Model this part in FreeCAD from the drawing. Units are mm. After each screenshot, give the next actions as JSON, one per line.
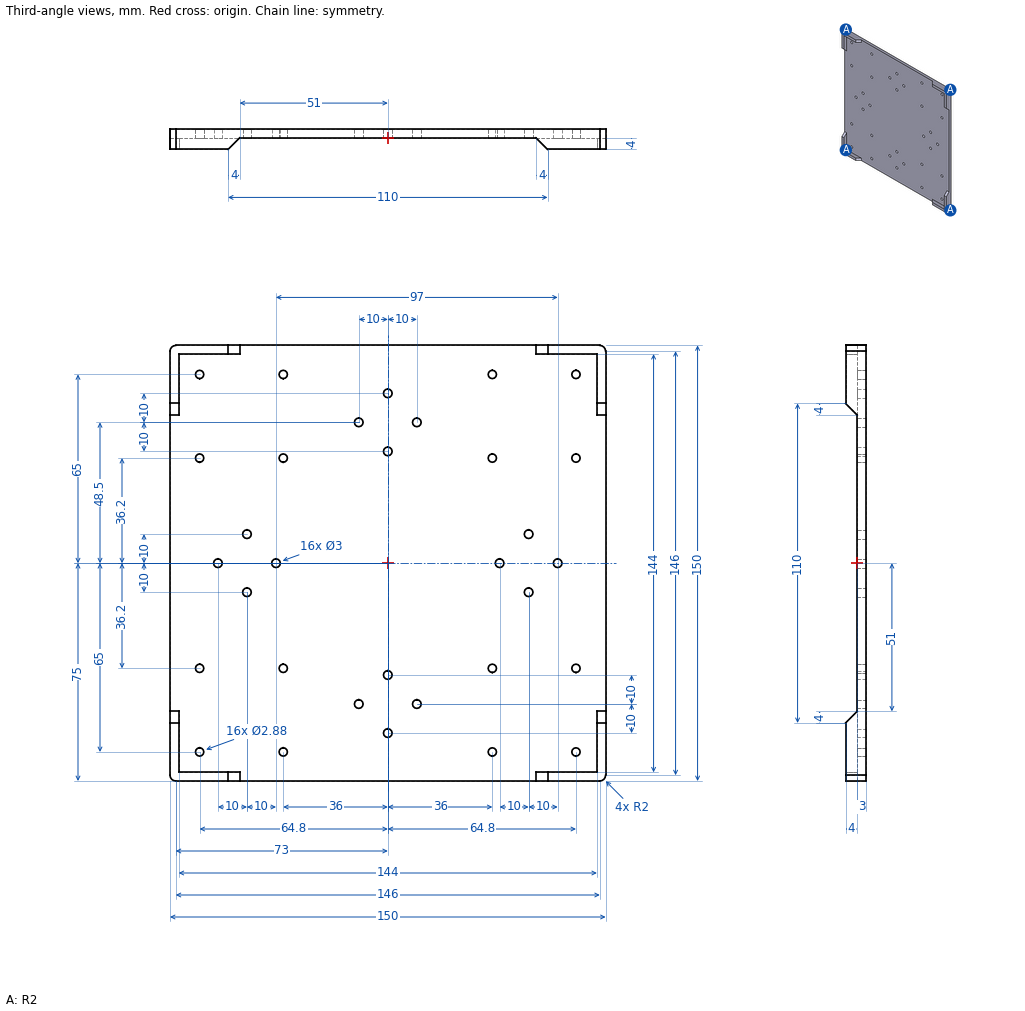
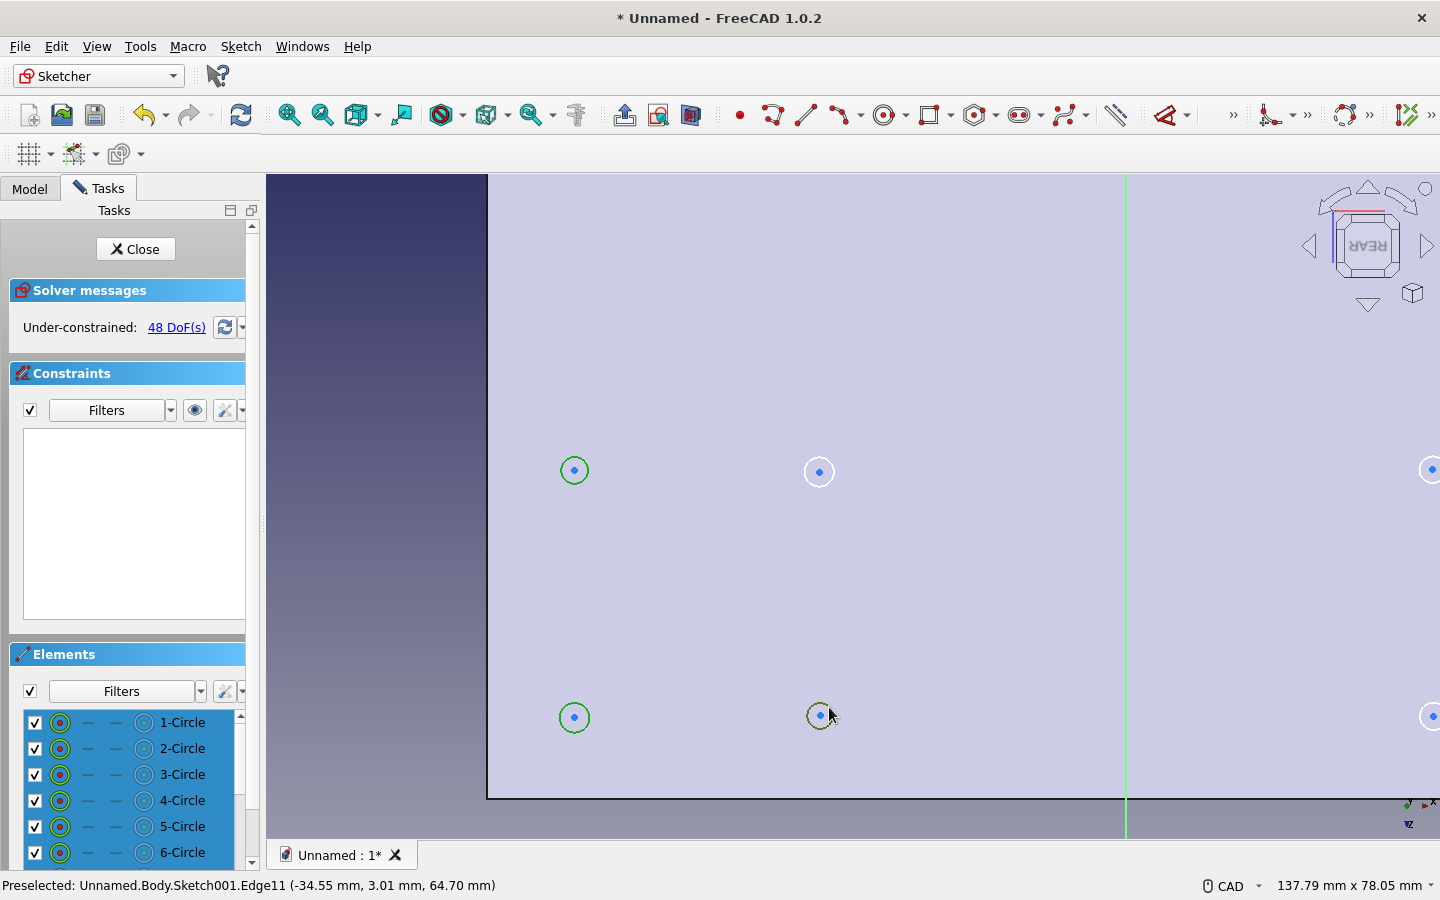
{"action": "left_click", "coordinate": [830, 462]}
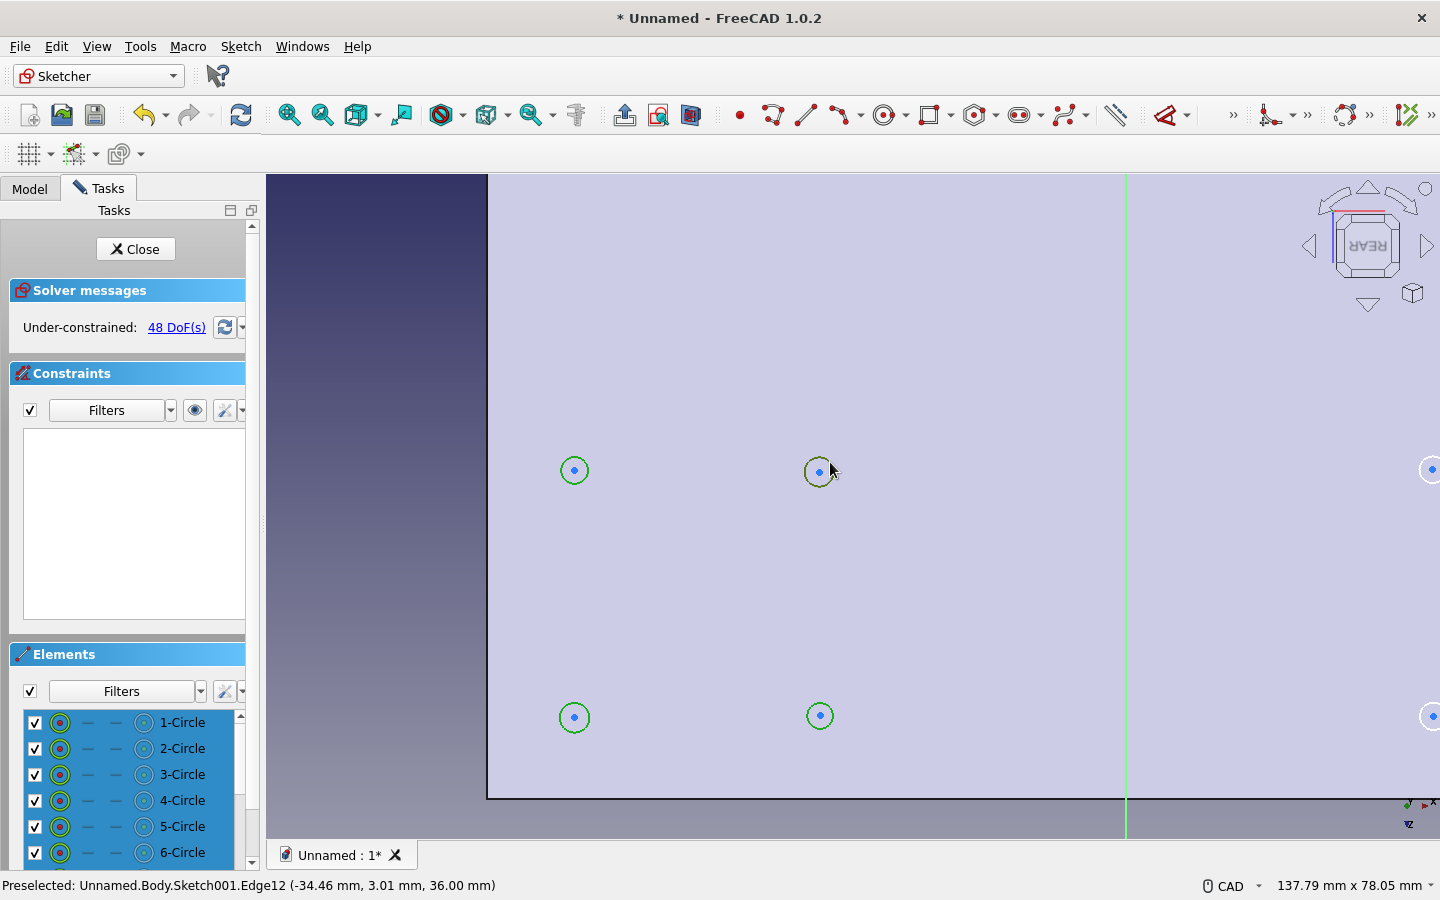
{"action": "scroll", "coordinate": [585, 708], "scroll_direction": "down", "scroll_amount": 5}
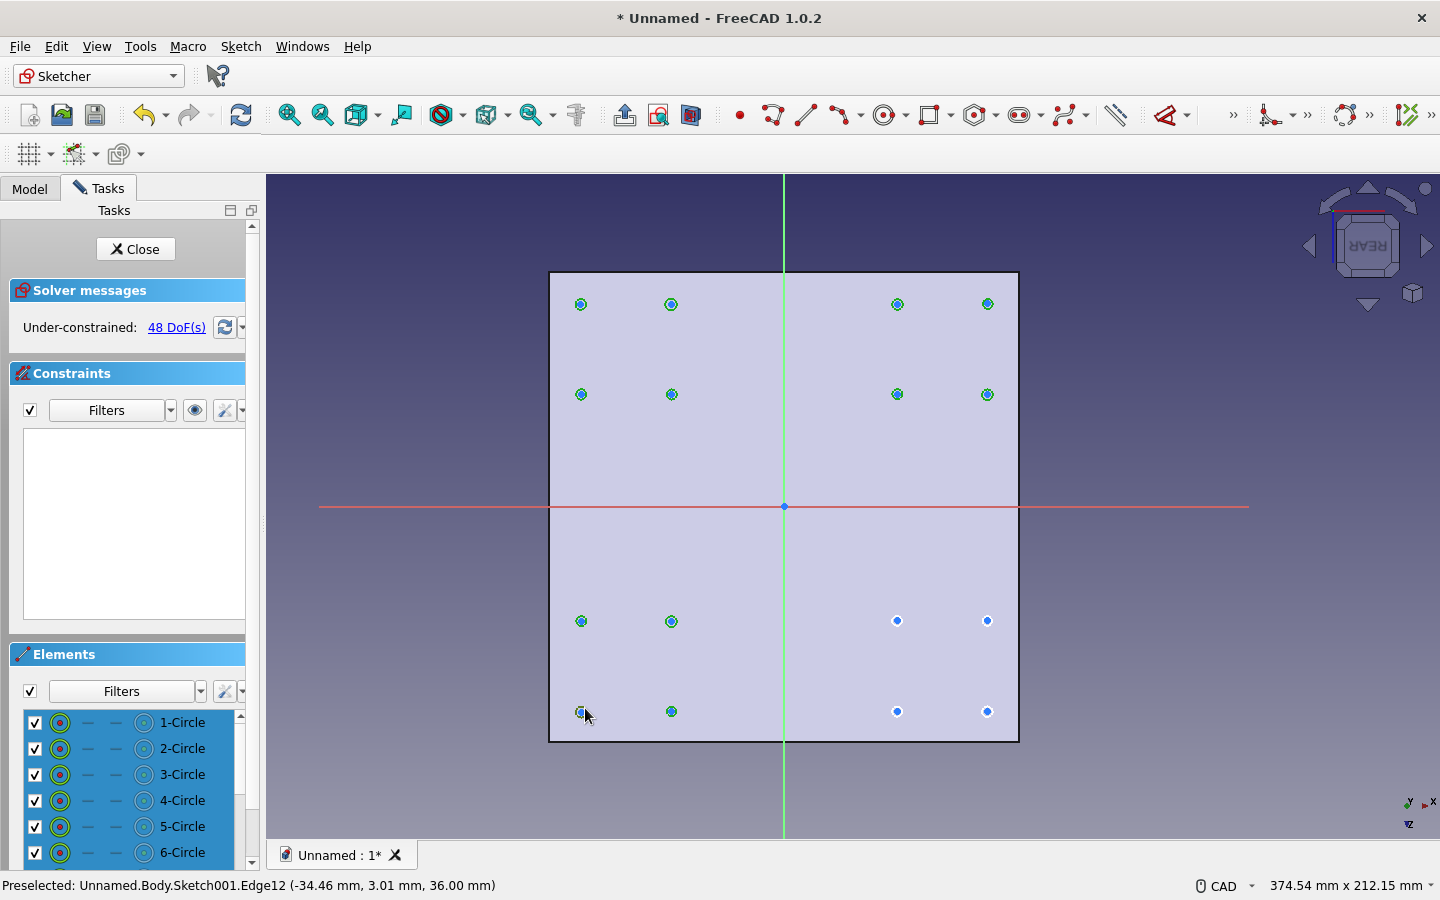
{"action": "scroll", "coordinate": [991, 708], "scroll_direction": "up", "scroll_amount": 5}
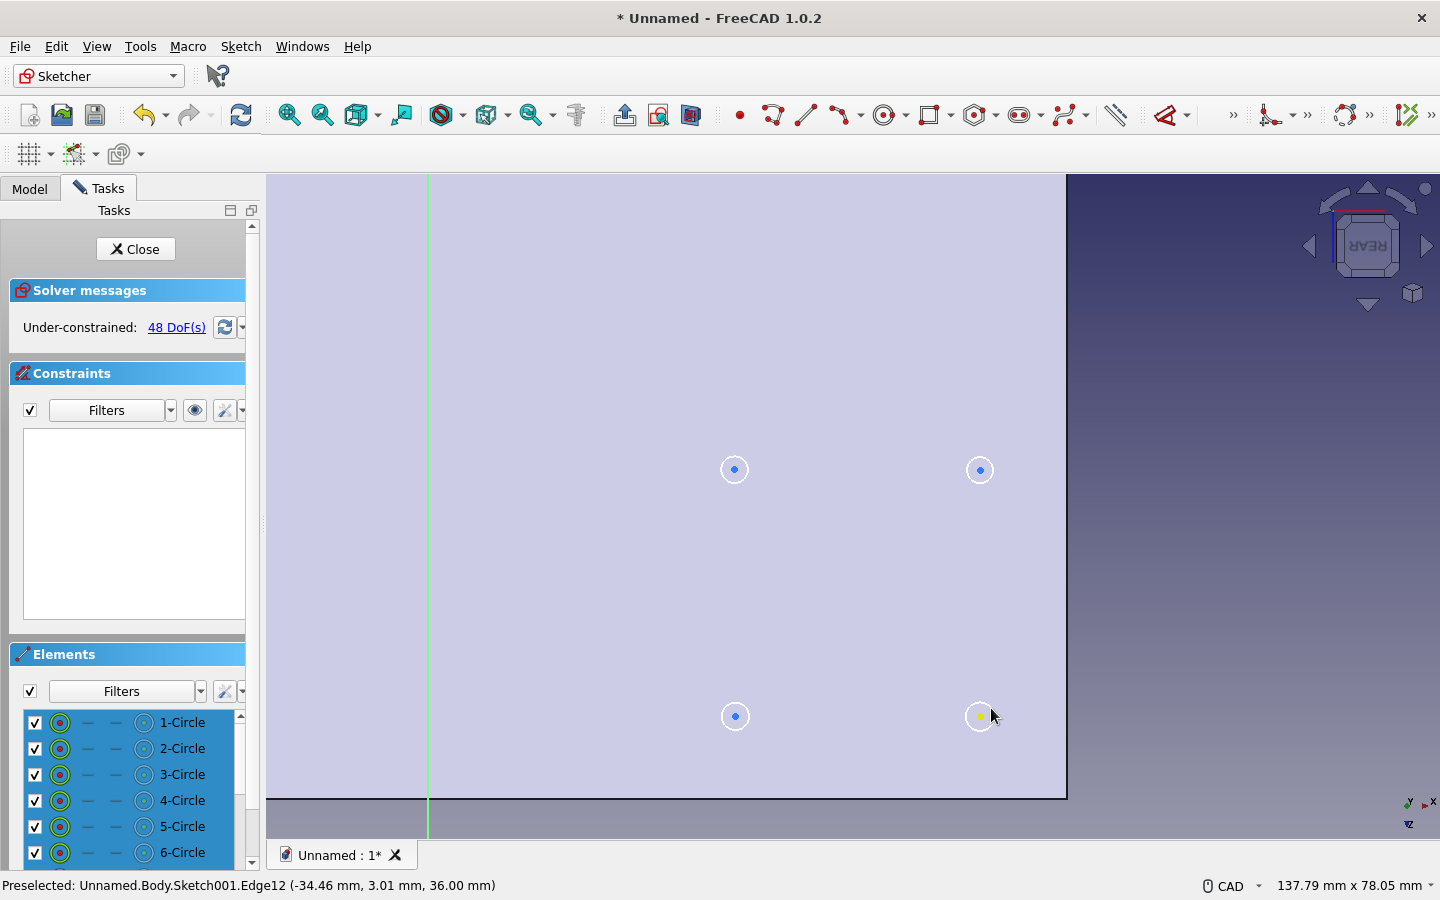
{"action": "left_click", "coordinate": [990, 707]}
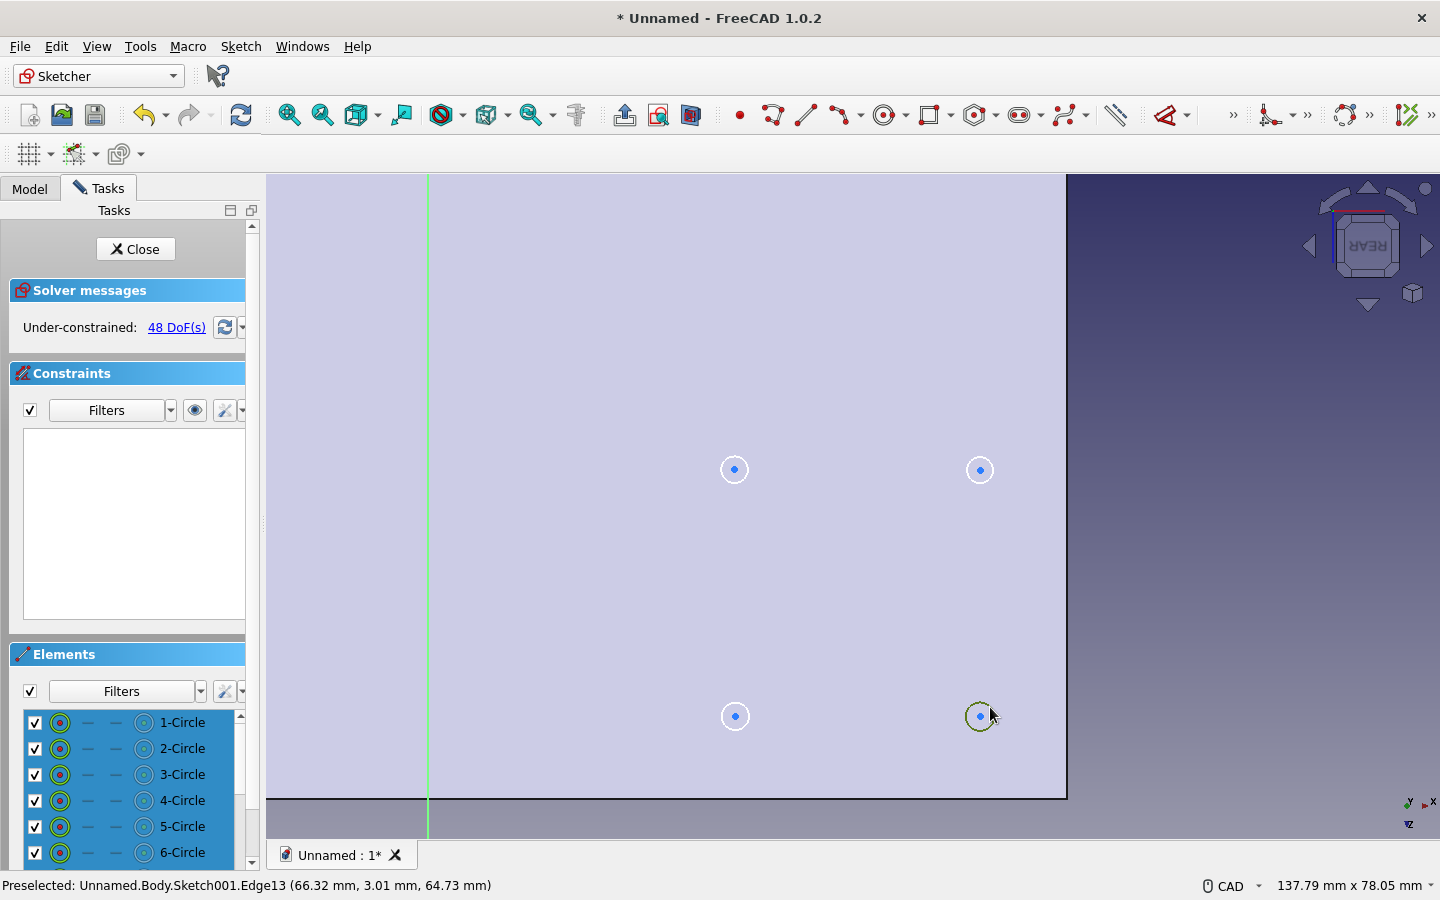
{"action": "left_click", "coordinate": [745, 707]}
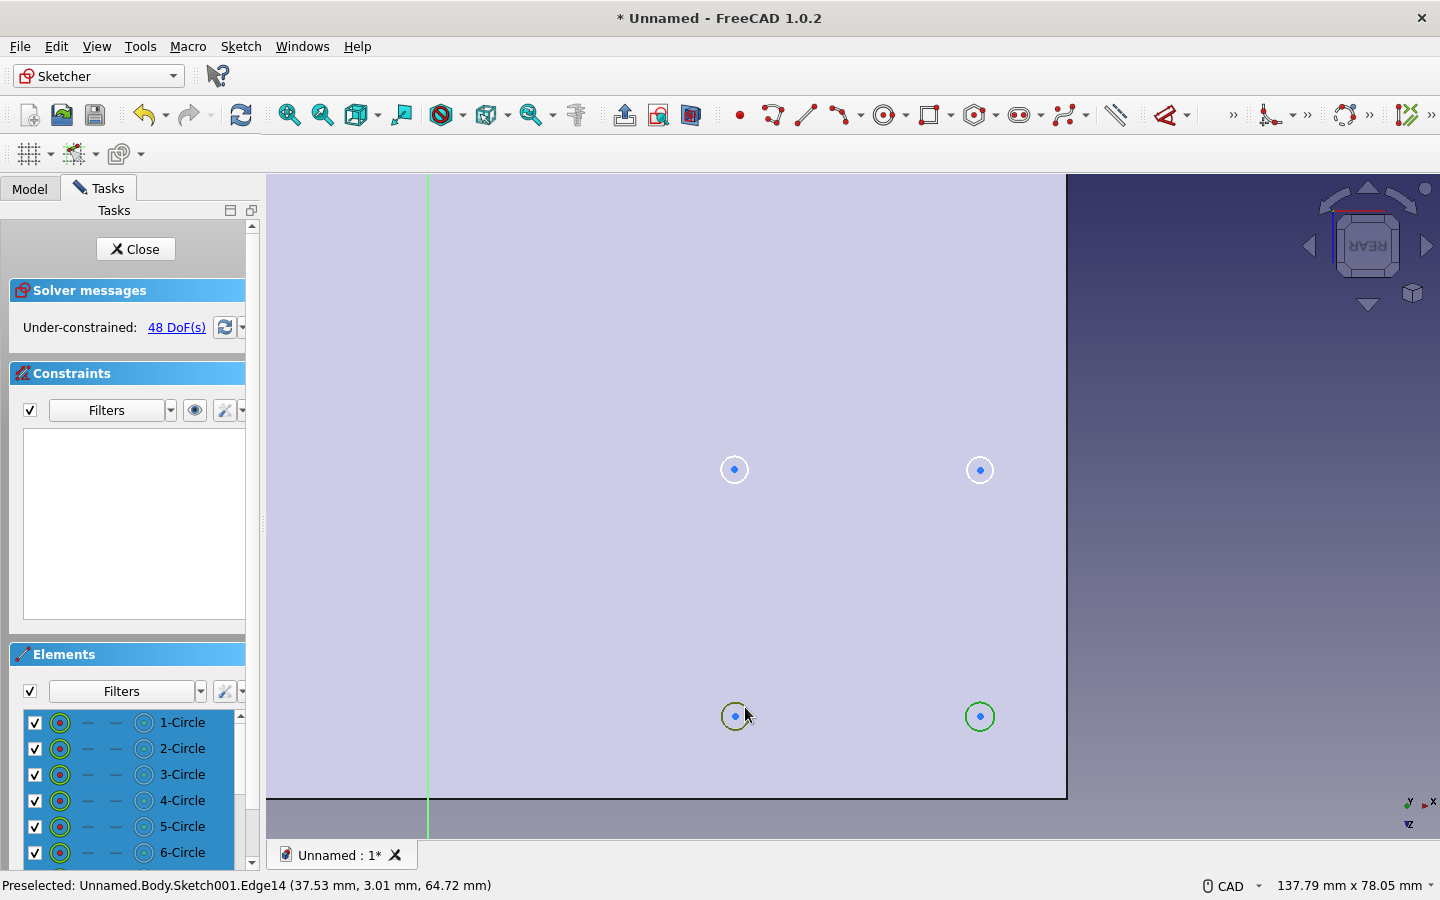
{"action": "left_click", "coordinate": [744, 460]}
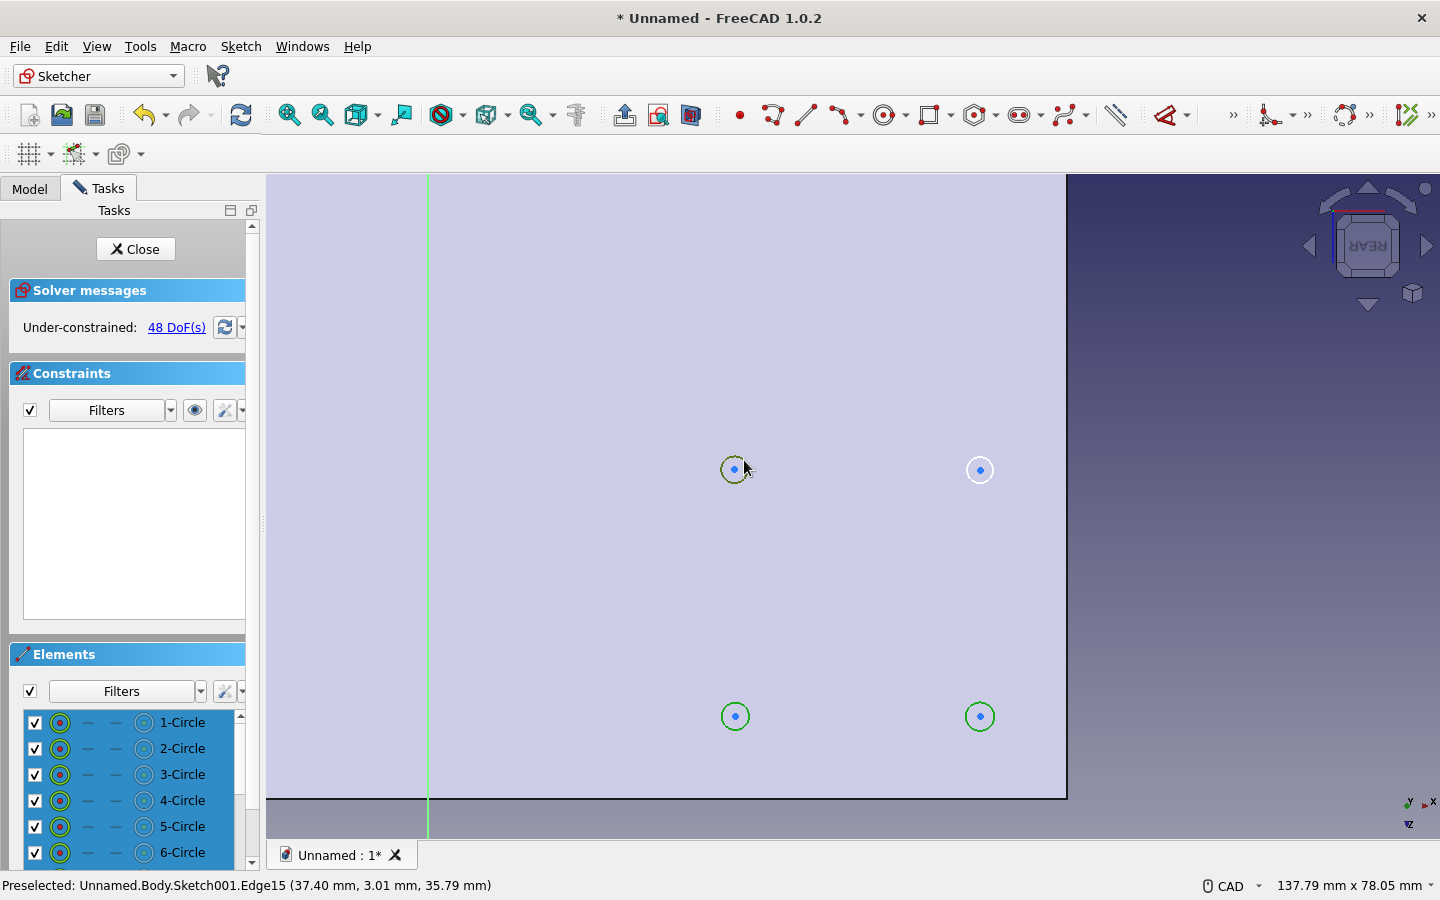
{"action": "left_click", "coordinate": [989, 461]}